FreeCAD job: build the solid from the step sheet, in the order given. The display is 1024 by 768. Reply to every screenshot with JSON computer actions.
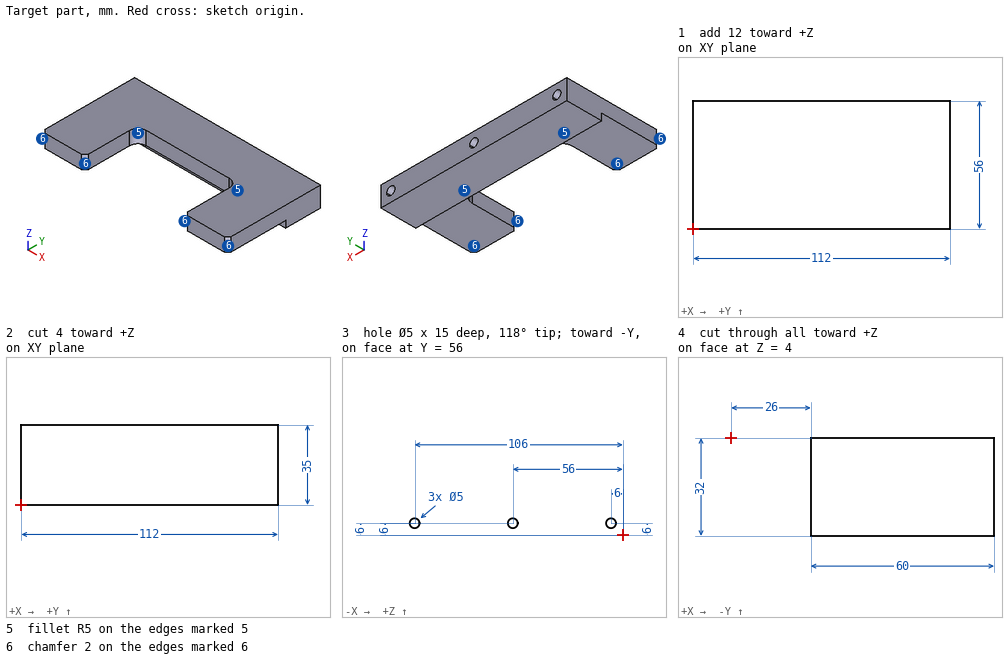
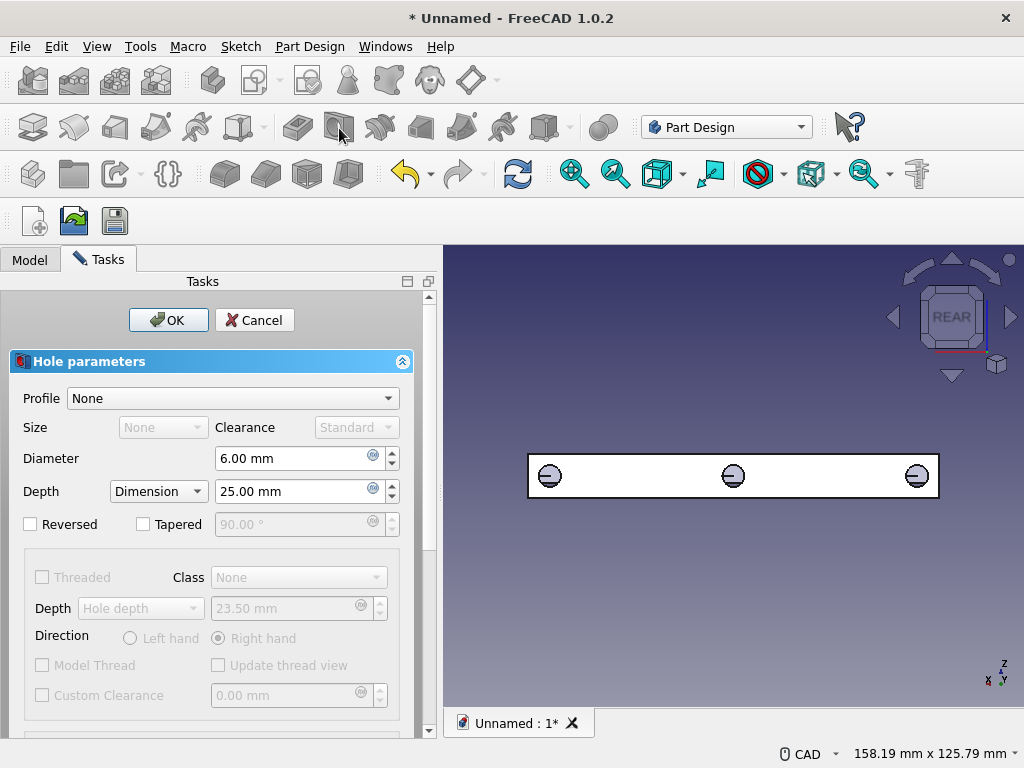
{"action": "triple_click", "coordinate": [300, 458]}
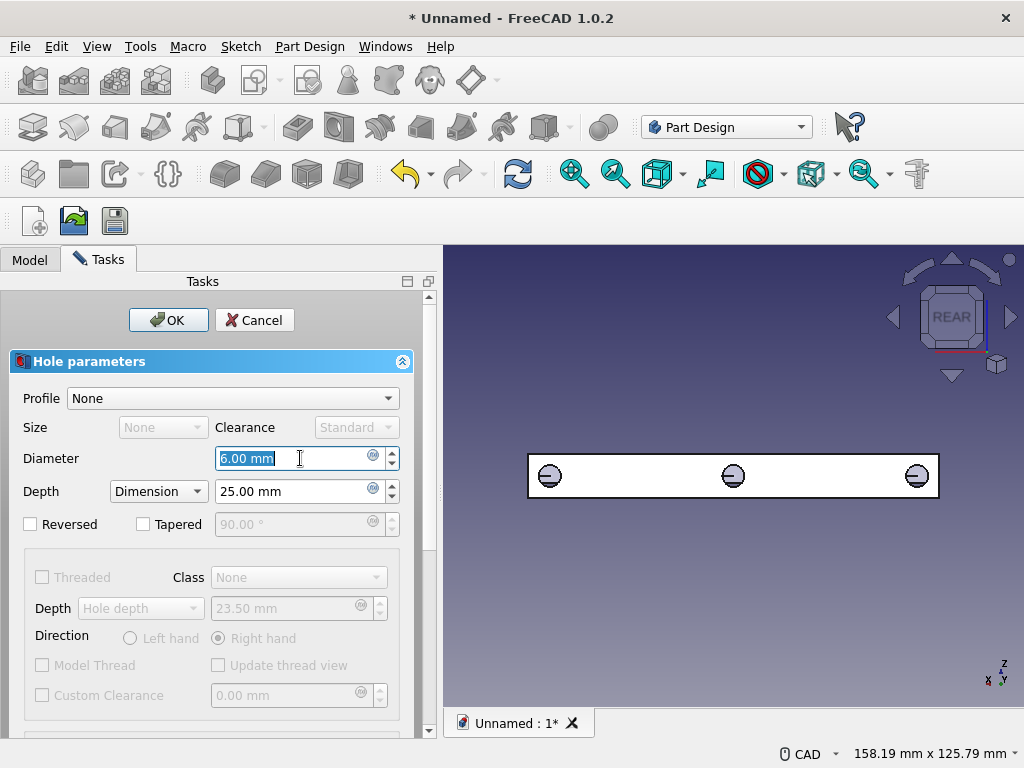
{"action": "type", "text": "5"}
{"action": "key", "text": "Tab"}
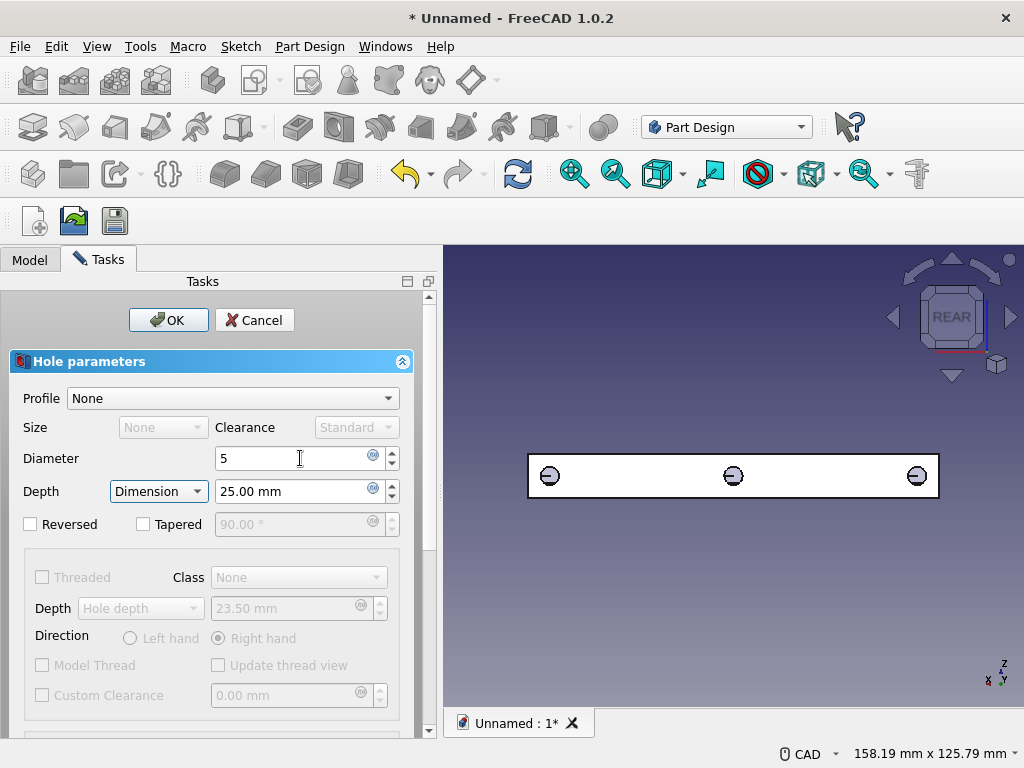
{"action": "triple_click", "coordinate": [300, 492]}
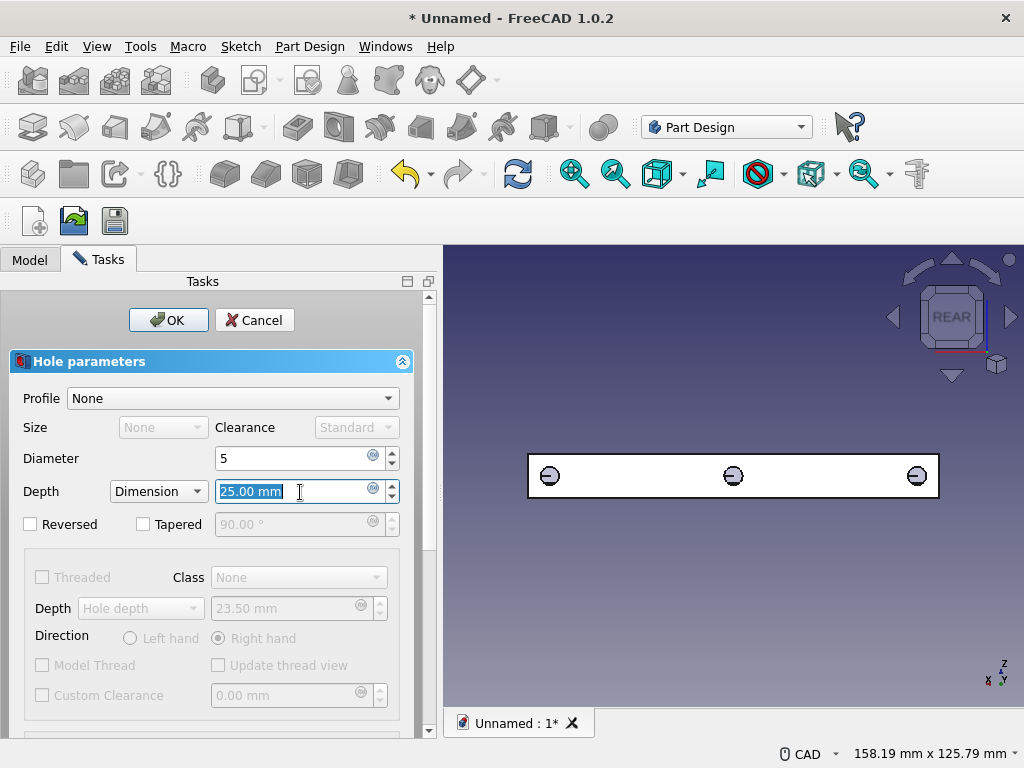
{"action": "type", "text": "15"}
{"action": "key", "text": "Tab"}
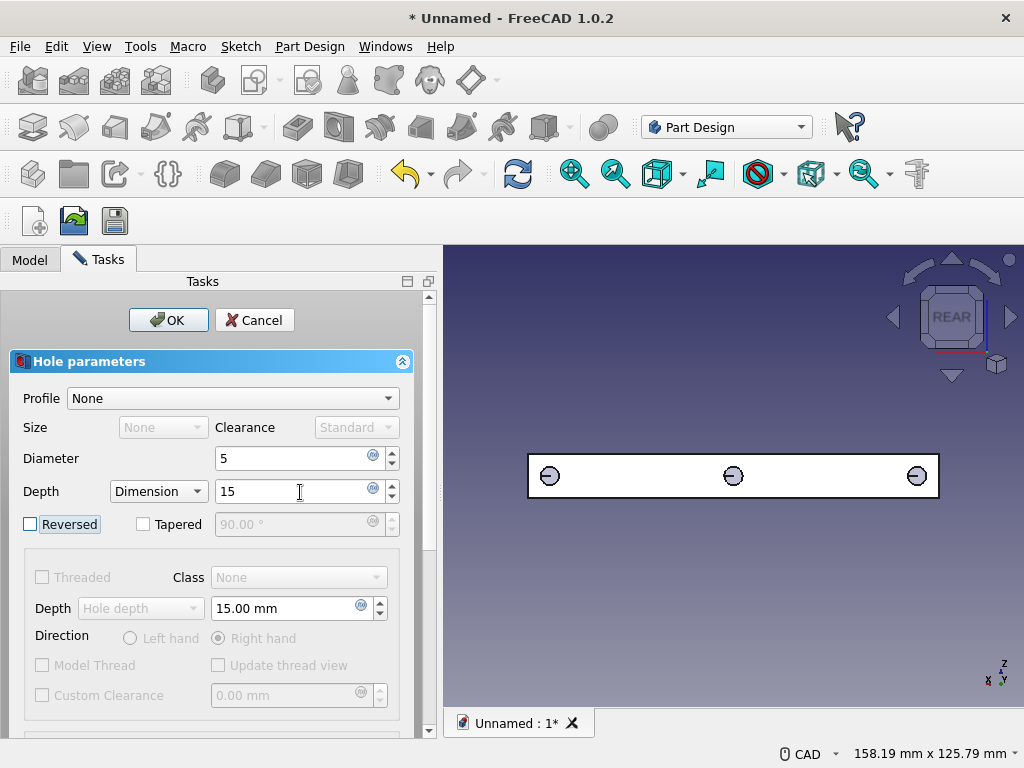
{"action": "left_click", "coordinate": [169, 320]}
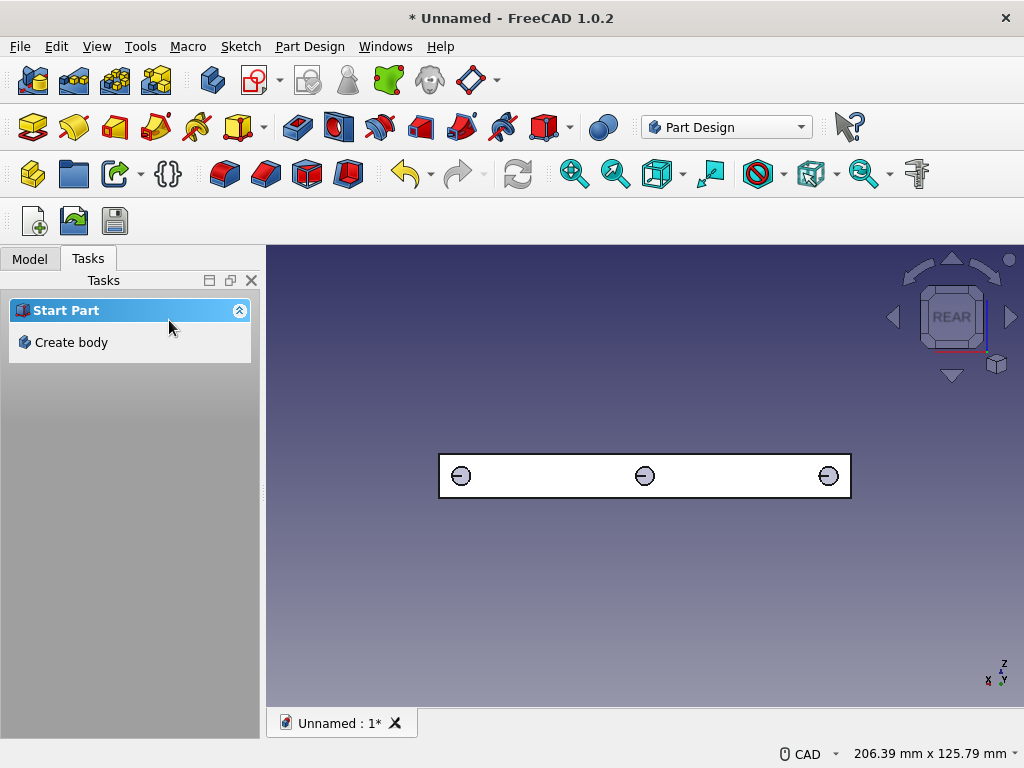
{"action": "key", "text": "5"}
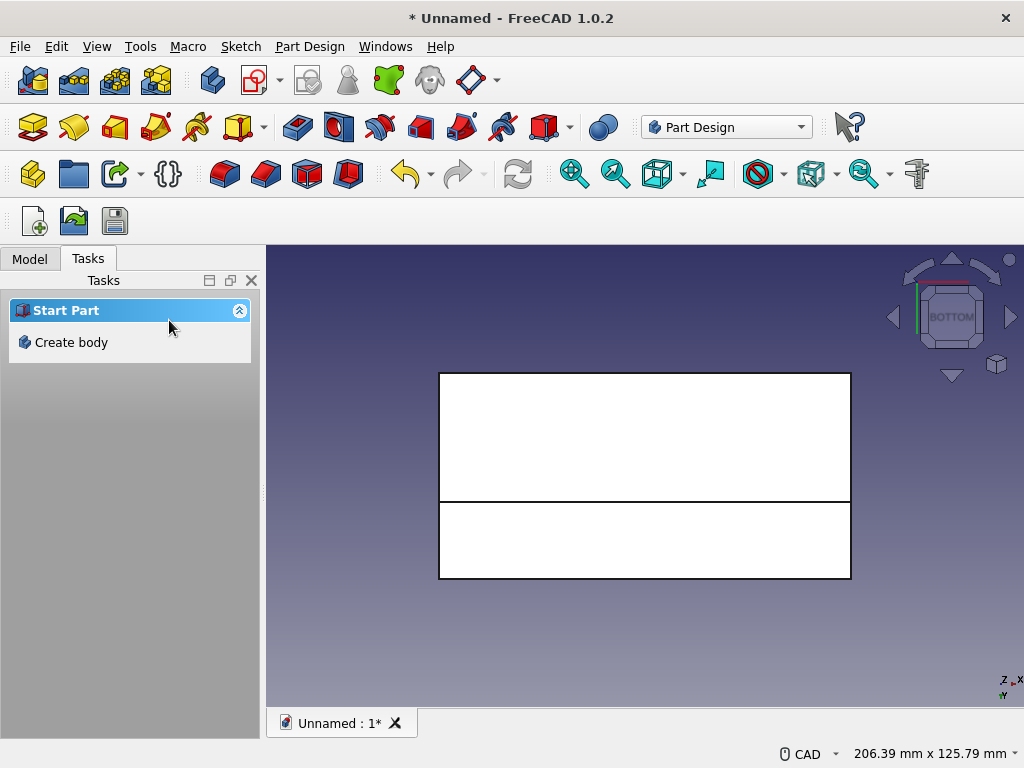
{"action": "left_click", "coordinate": [763, 436]}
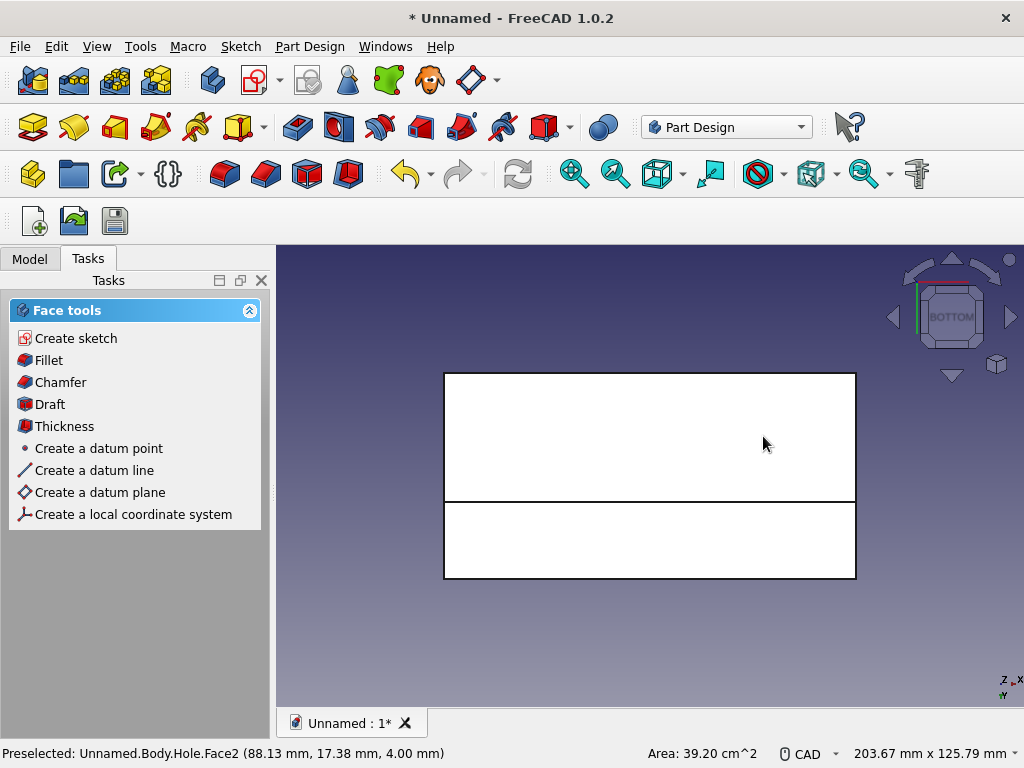
{"action": "left_click", "coordinate": [254, 80]}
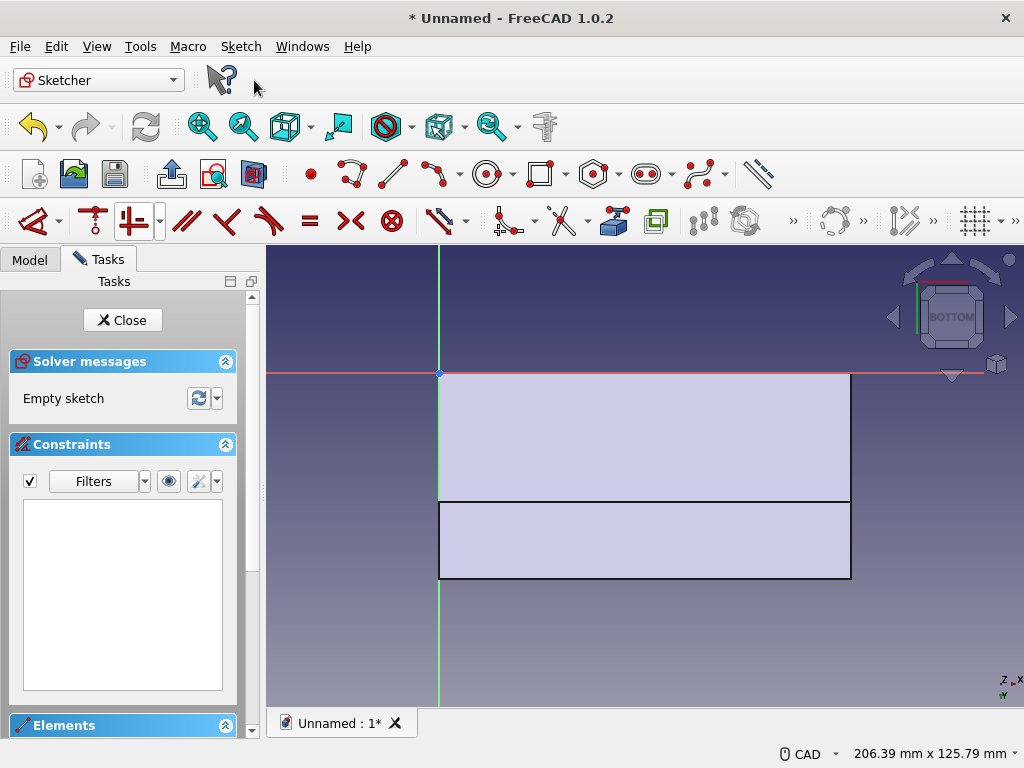
{"action": "left_click", "coordinate": [540, 174]}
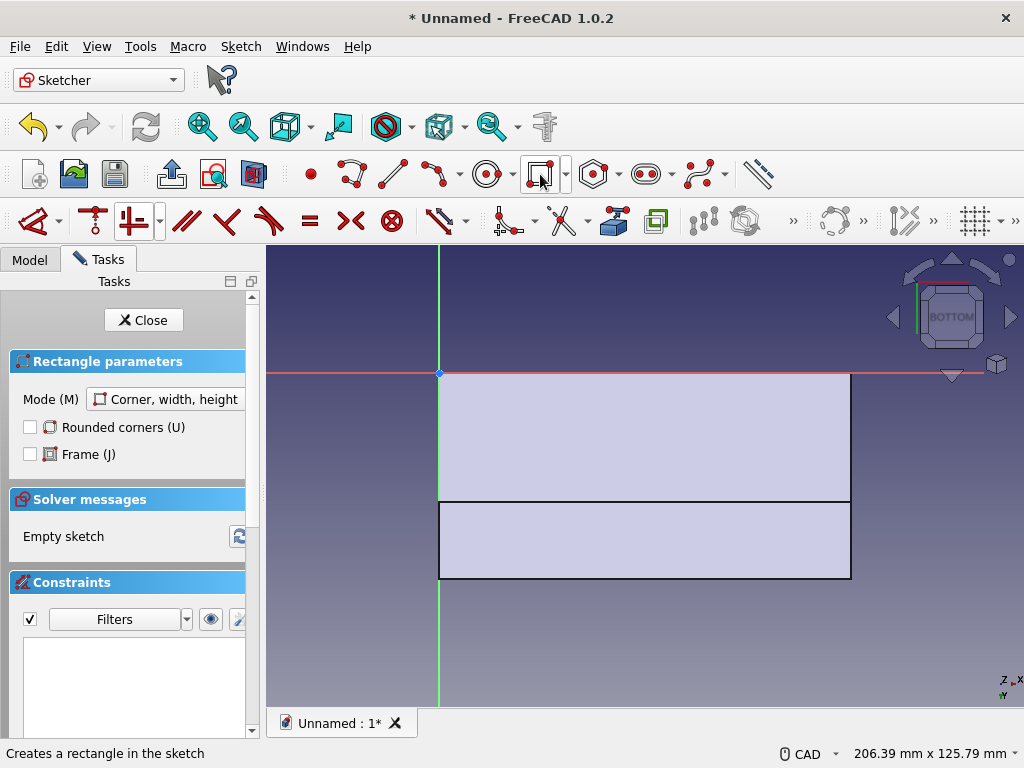
{"action": "left_click", "coordinate": [535, 373]}
{"action": "left_click", "coordinate": [755, 491]}
{"action": "key", "text": "Escape"}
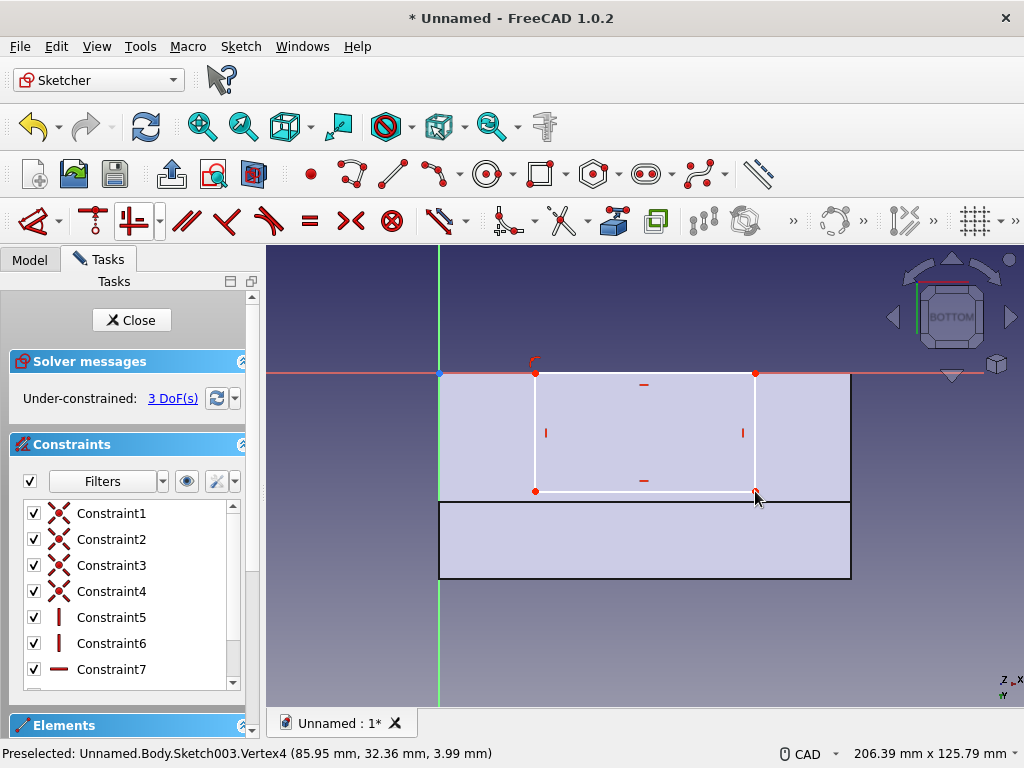
{"action": "left_click", "coordinate": [32, 222]}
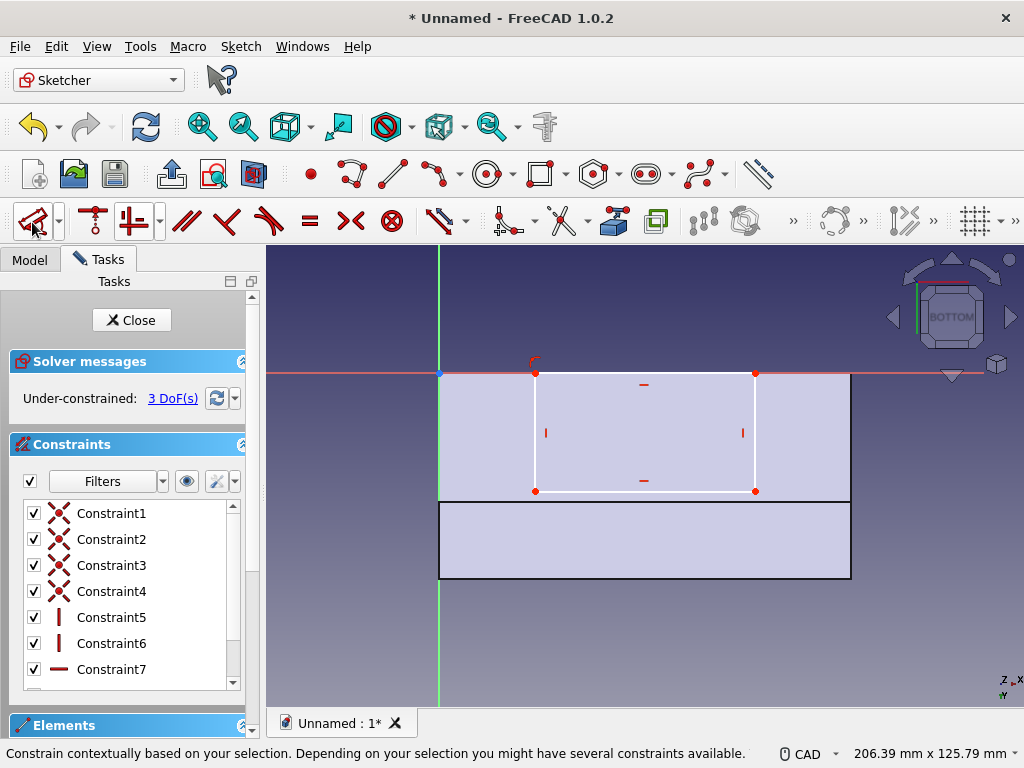
{"action": "left_click", "coordinate": [535, 409]}
{"action": "left_click", "coordinate": [501, 433]}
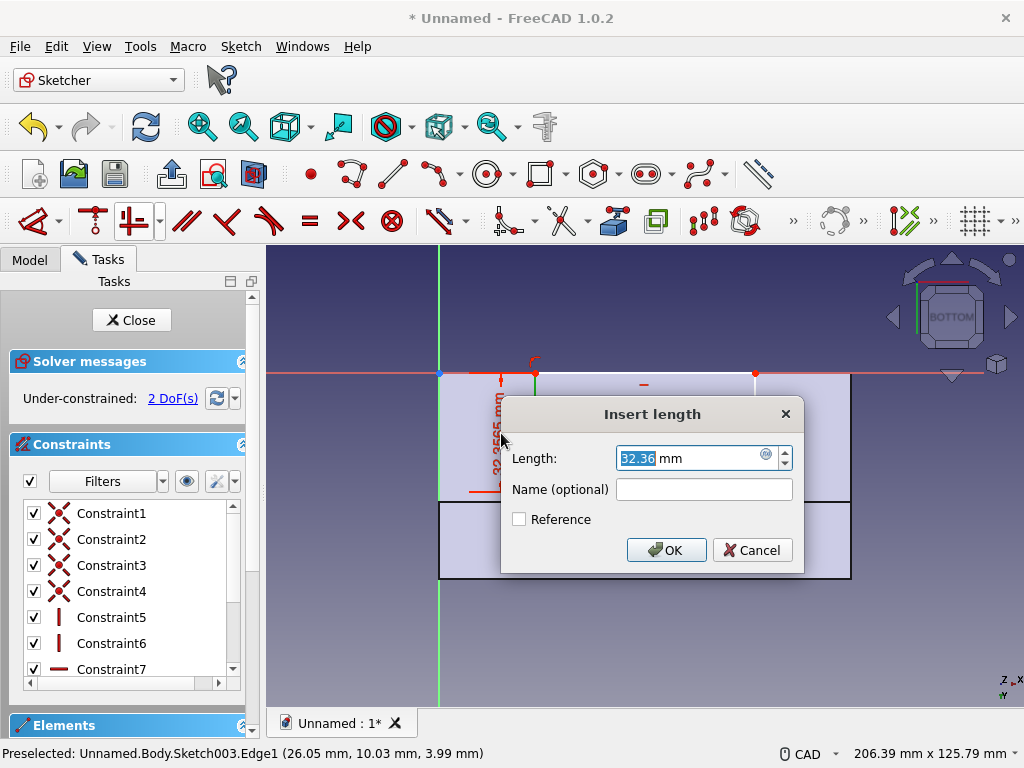
{"action": "type", "text": "32"}
{"action": "key", "text": "Return"}